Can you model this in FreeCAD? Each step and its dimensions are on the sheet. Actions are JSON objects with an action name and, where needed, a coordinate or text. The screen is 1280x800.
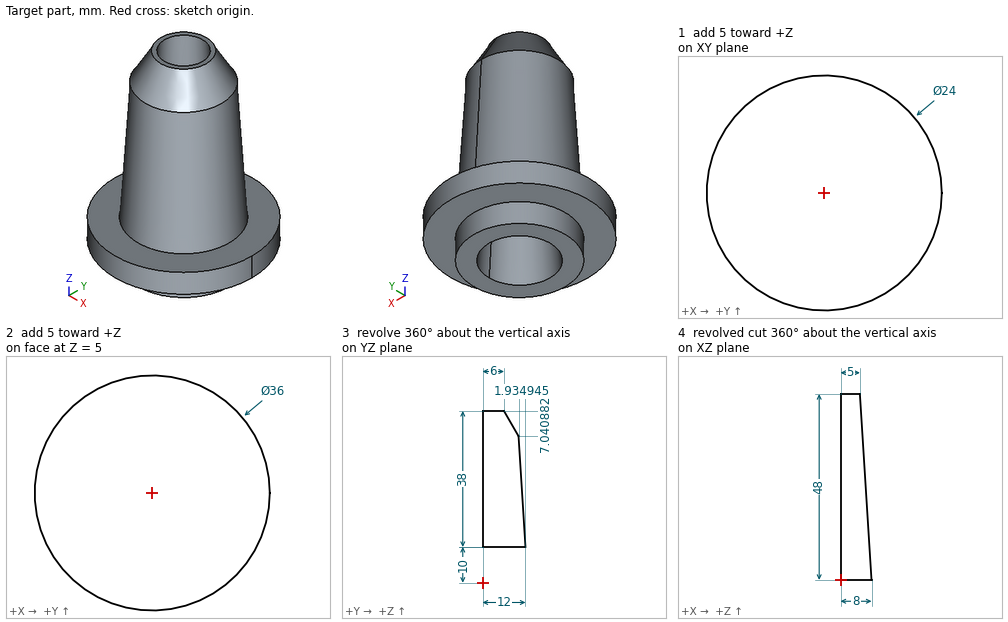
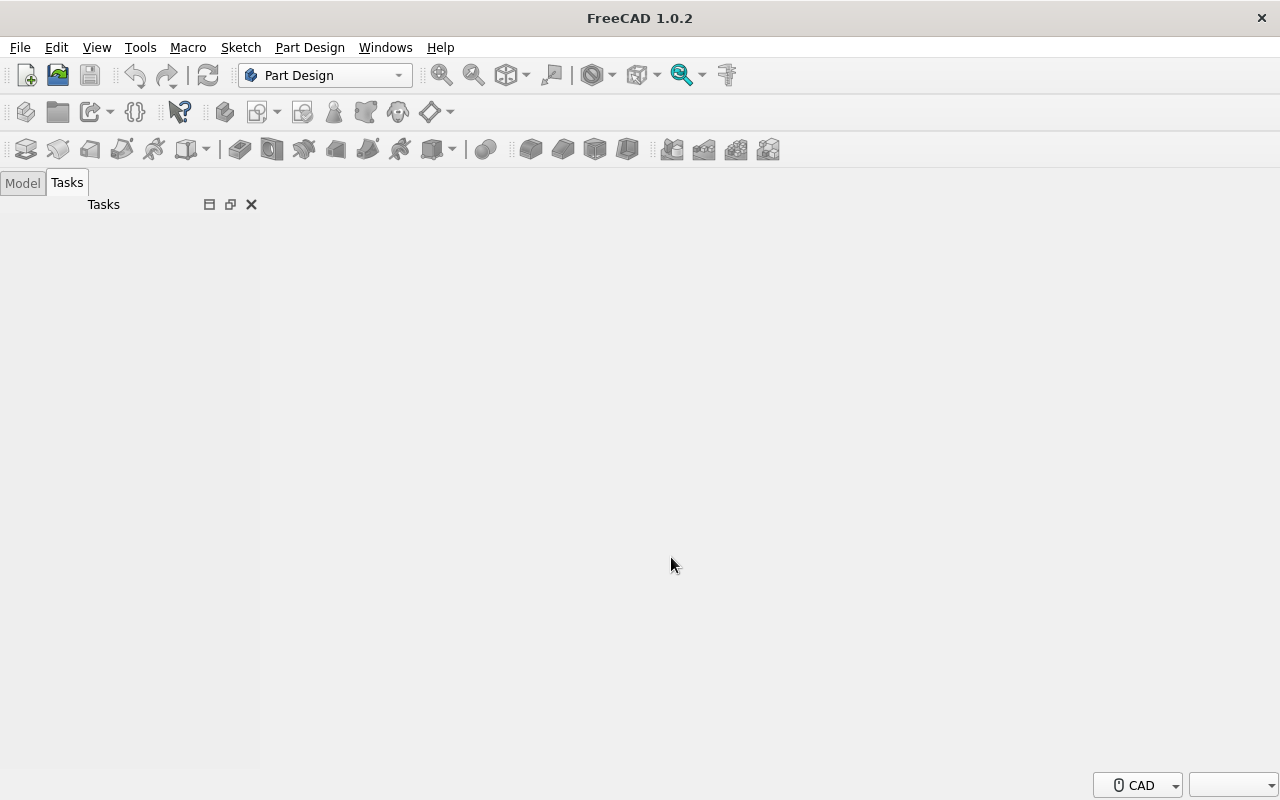
{"action": "left_click", "coordinate": [26, 76]}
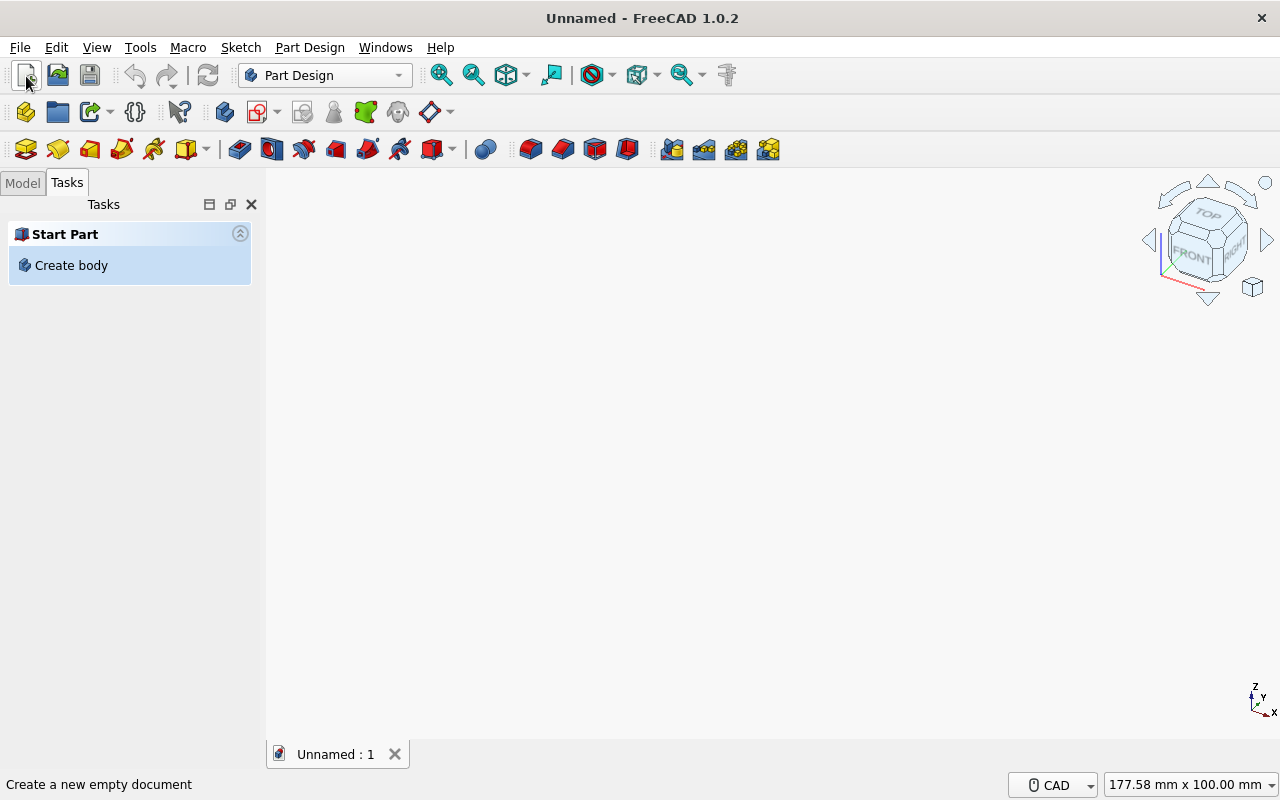
{"action": "left_click", "coordinate": [258, 112]}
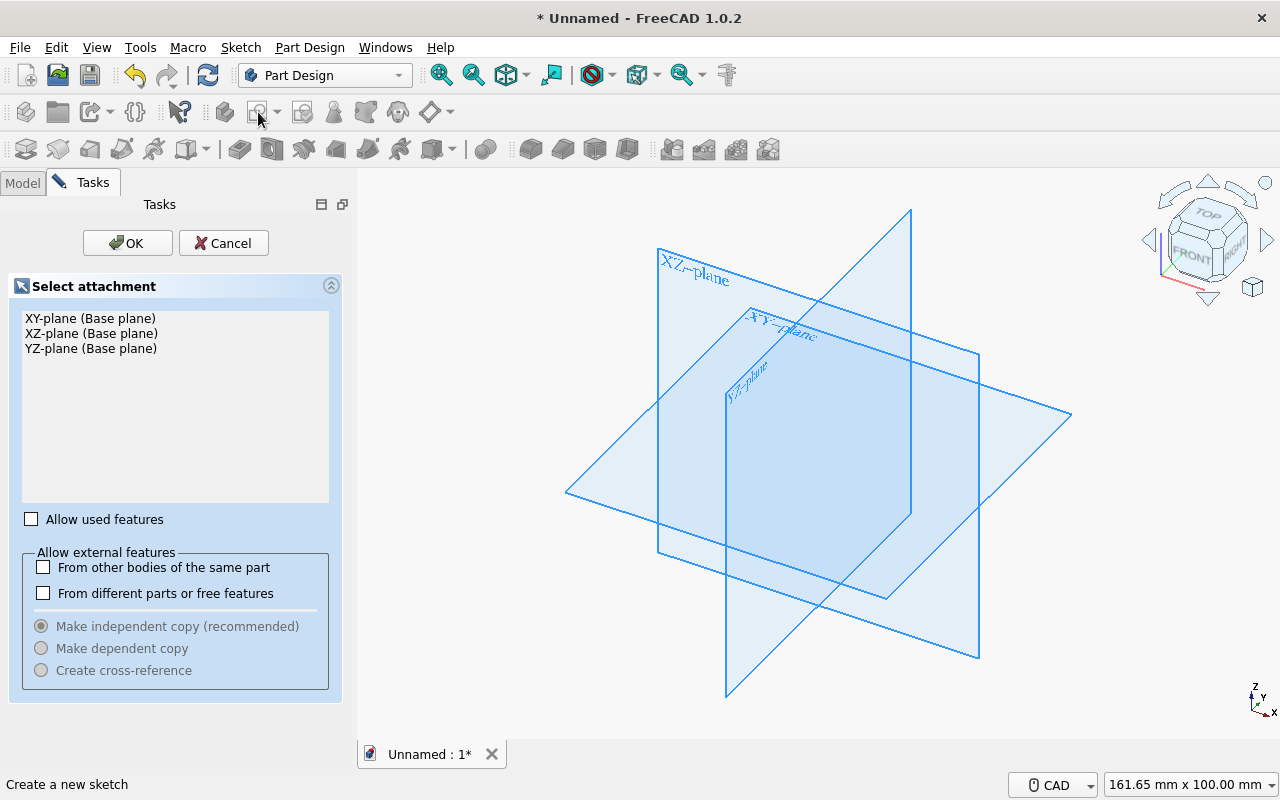
{"action": "left_click", "coordinate": [82, 318]}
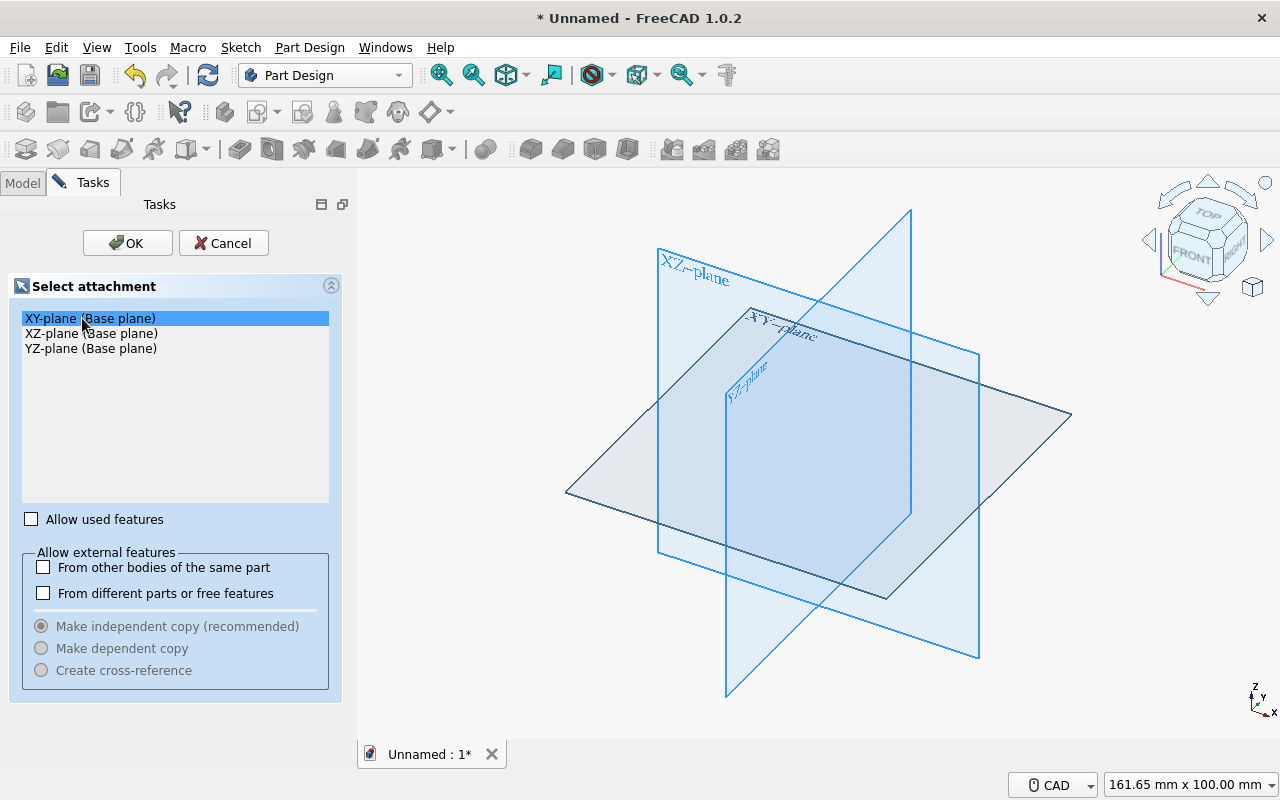
{"action": "left_click", "coordinate": [128, 243]}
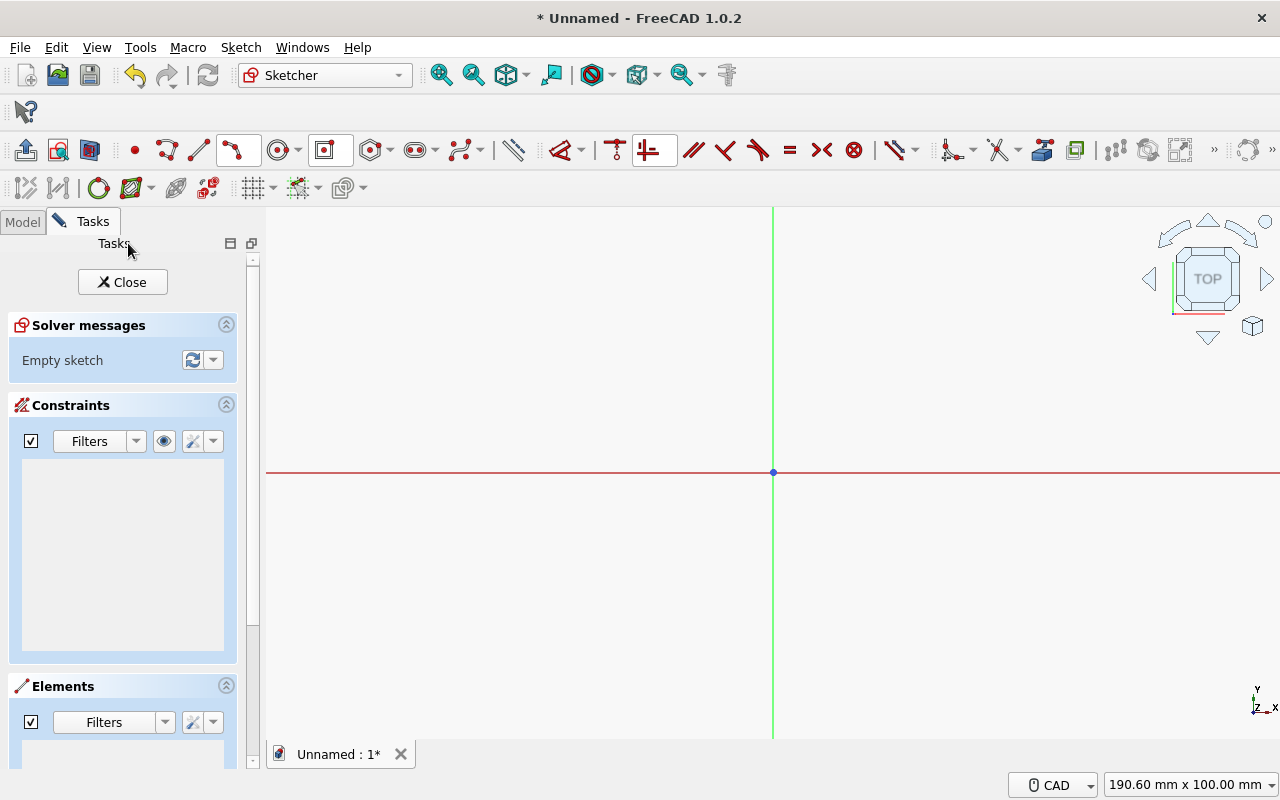
{"action": "scroll", "coordinate": [813, 473], "scroll_direction": "up", "scroll_amount": 5}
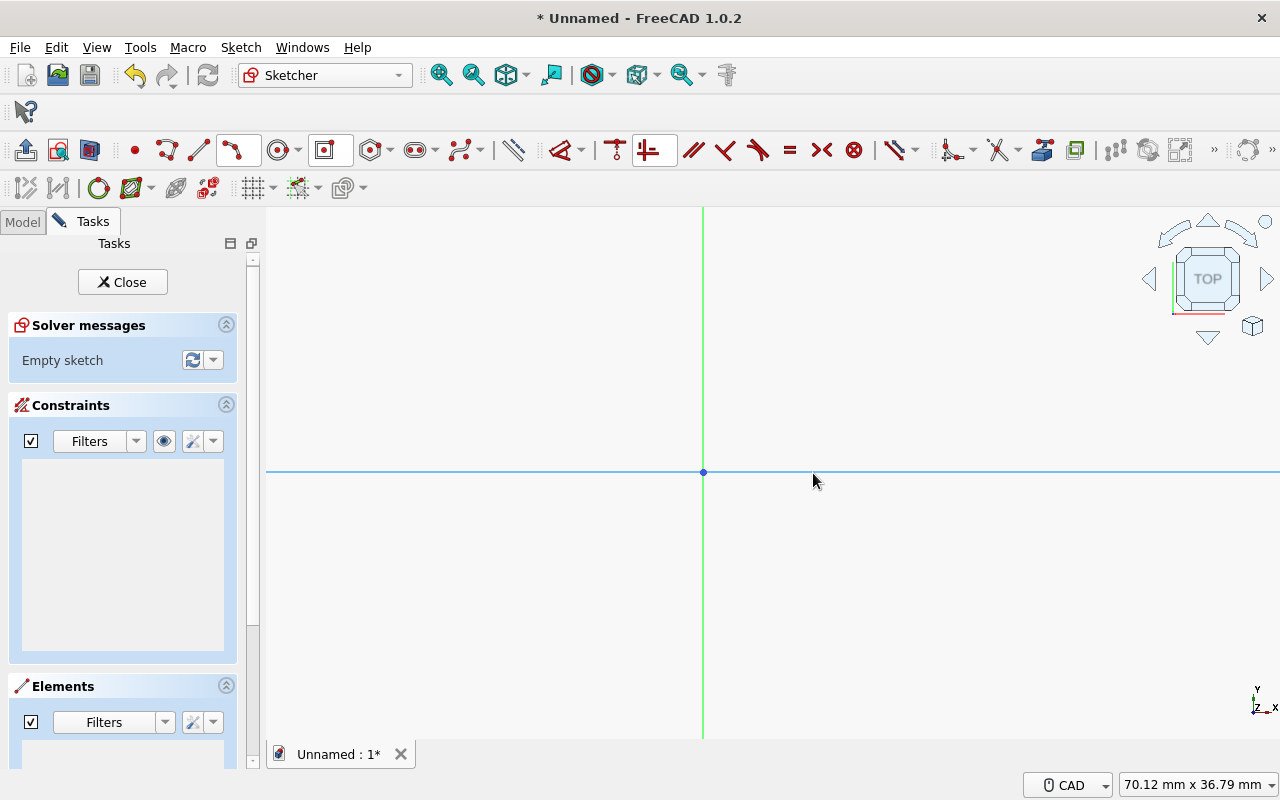
{"action": "left_click", "coordinate": [278, 150]}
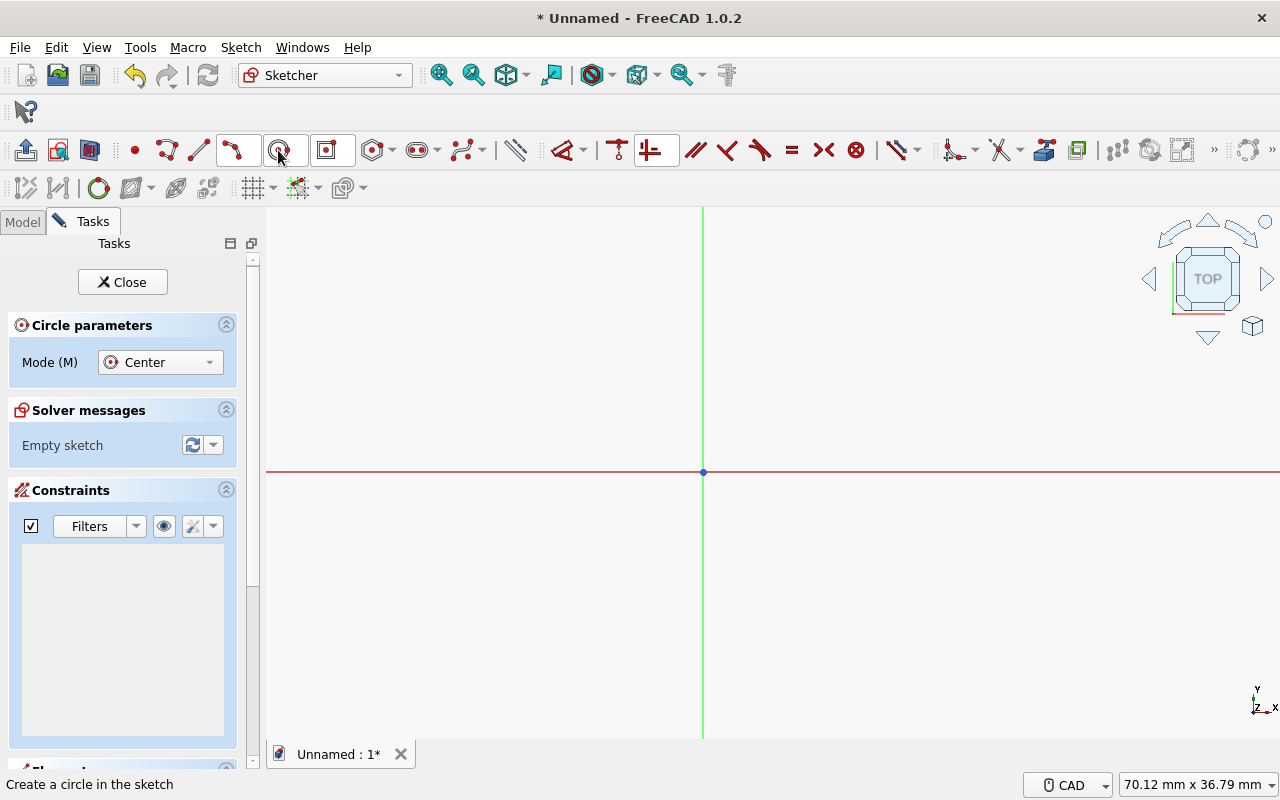
{"action": "left_click", "coordinate": [703, 472]}
{"action": "mouse_move", "coordinate": [826, 349]}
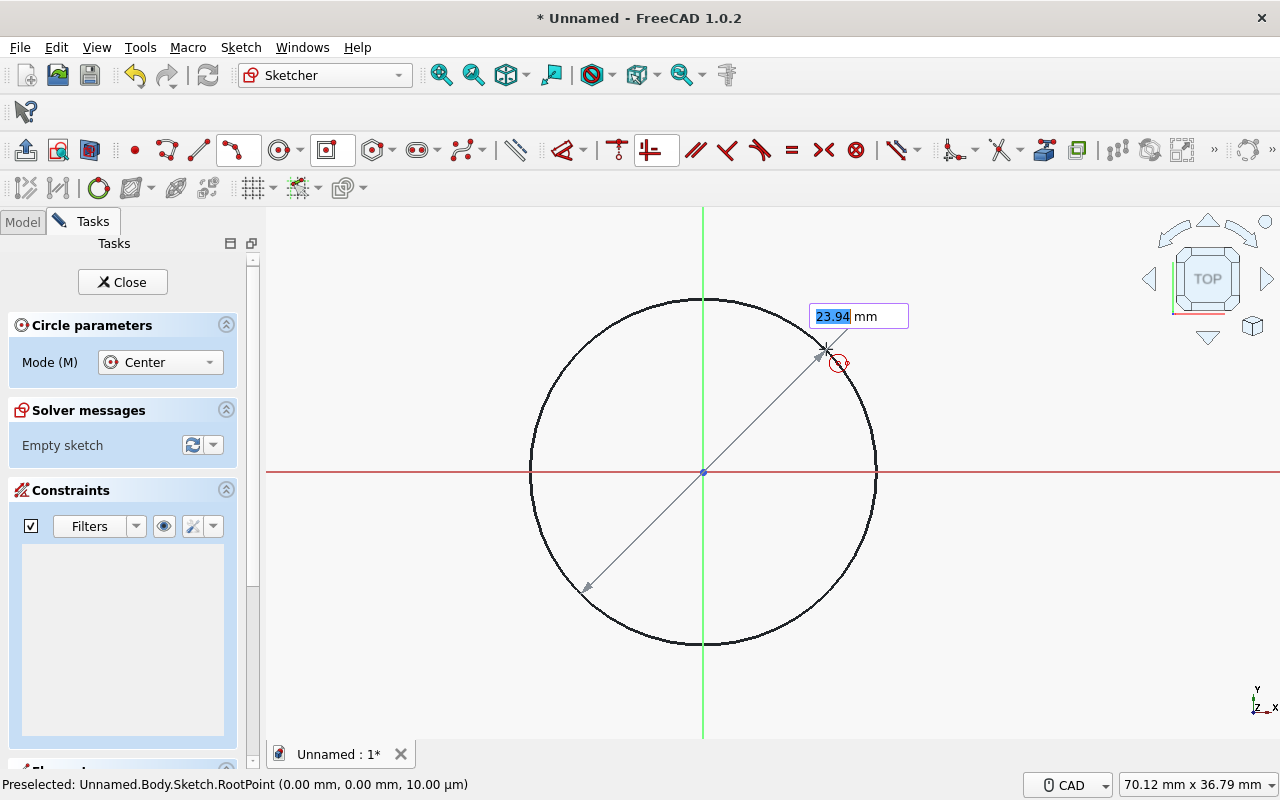
{"action": "type", "text": "24"}
{"action": "key", "text": "Return"}
{"action": "key", "text": "Escape"}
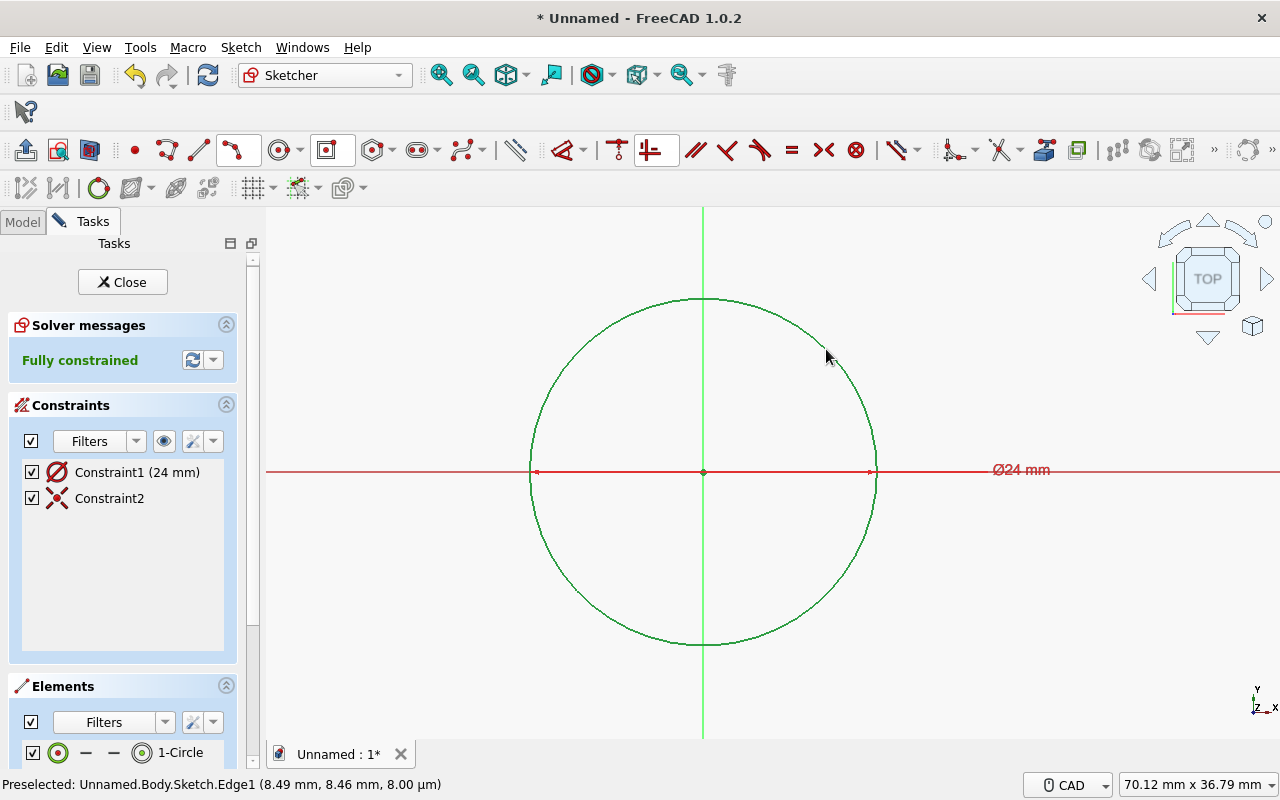
{"action": "left_click", "coordinate": [123, 282]}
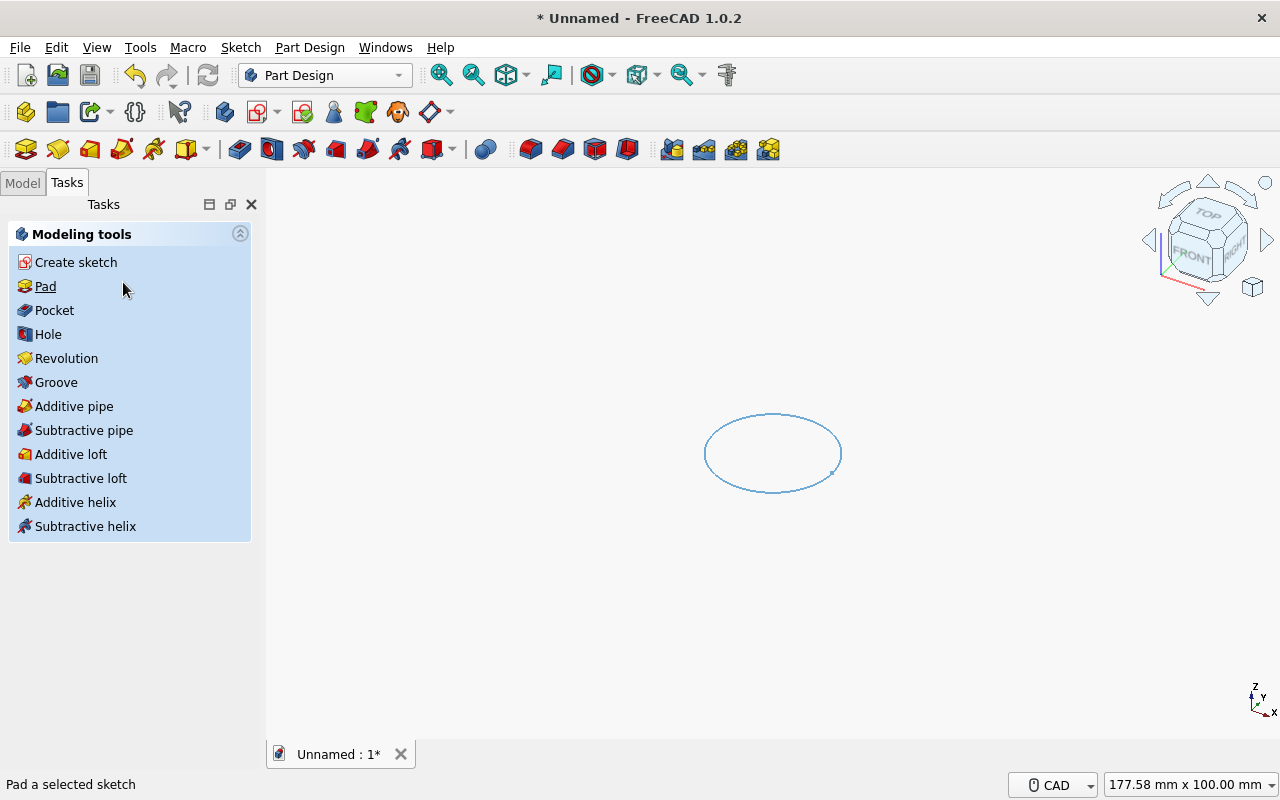
{"action": "left_click", "coordinate": [26, 150]}